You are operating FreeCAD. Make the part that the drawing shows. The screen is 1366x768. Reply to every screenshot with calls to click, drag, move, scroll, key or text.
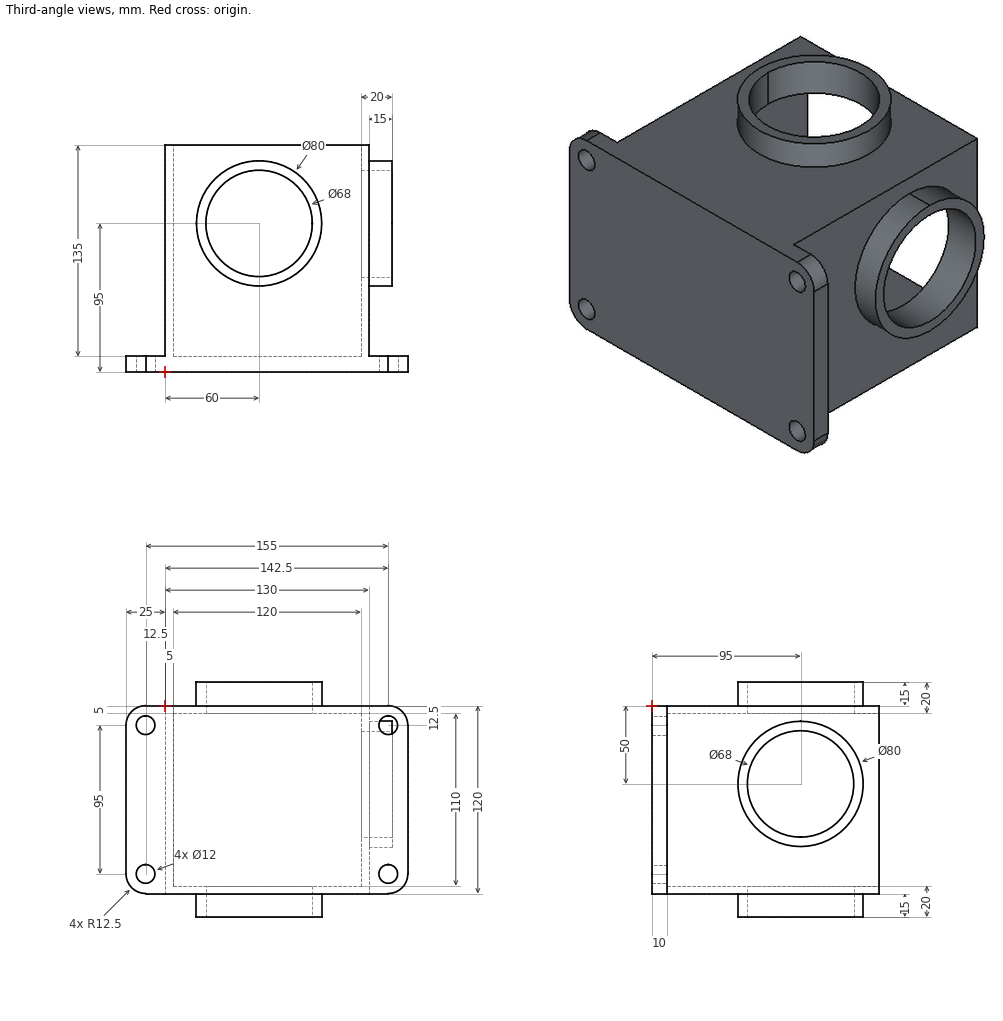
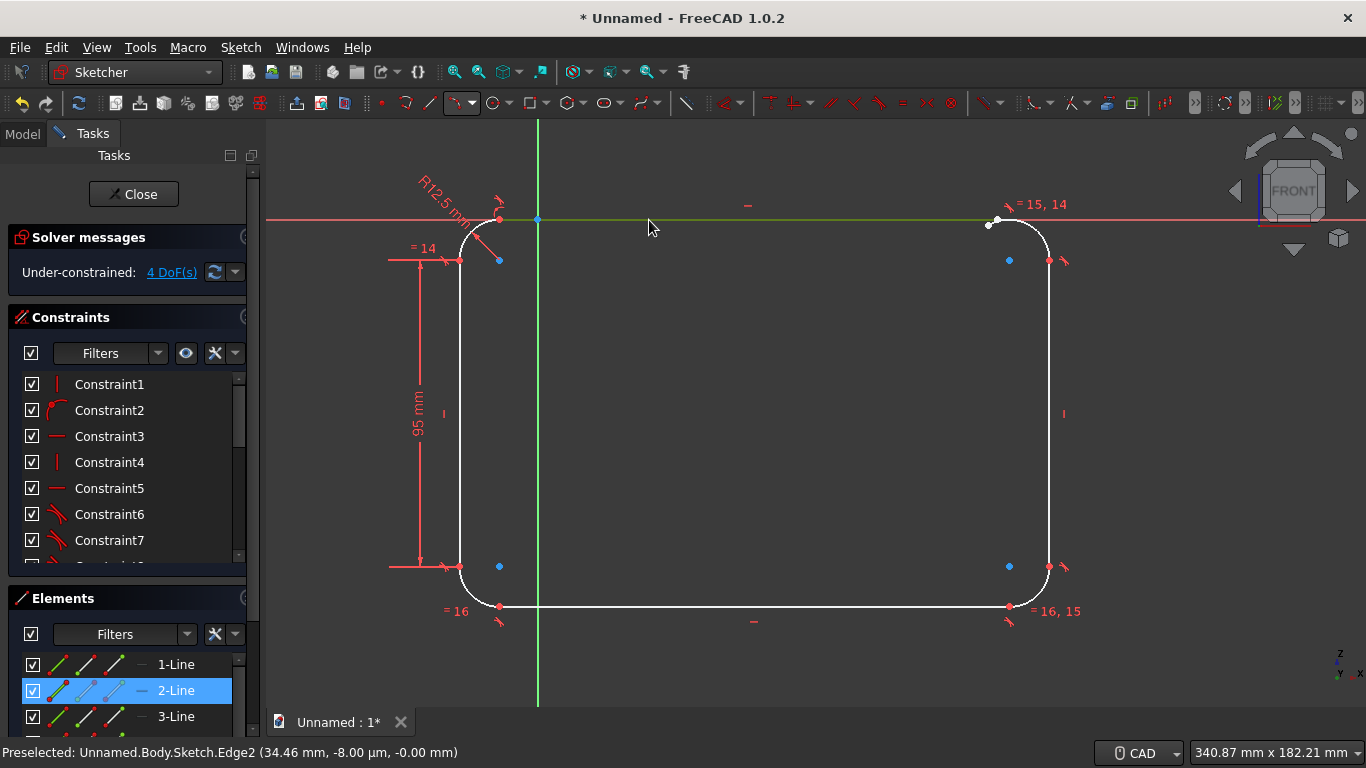
click(742, 104)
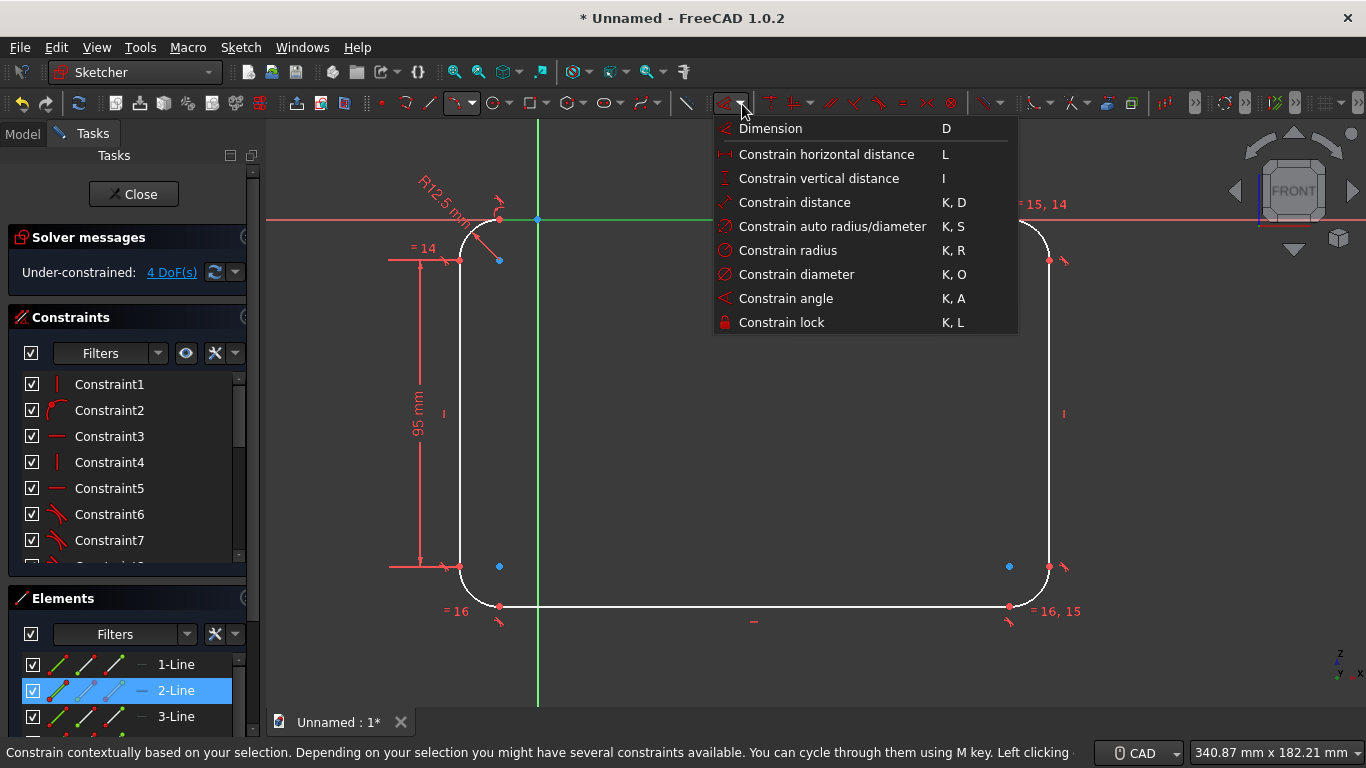
click(866, 154)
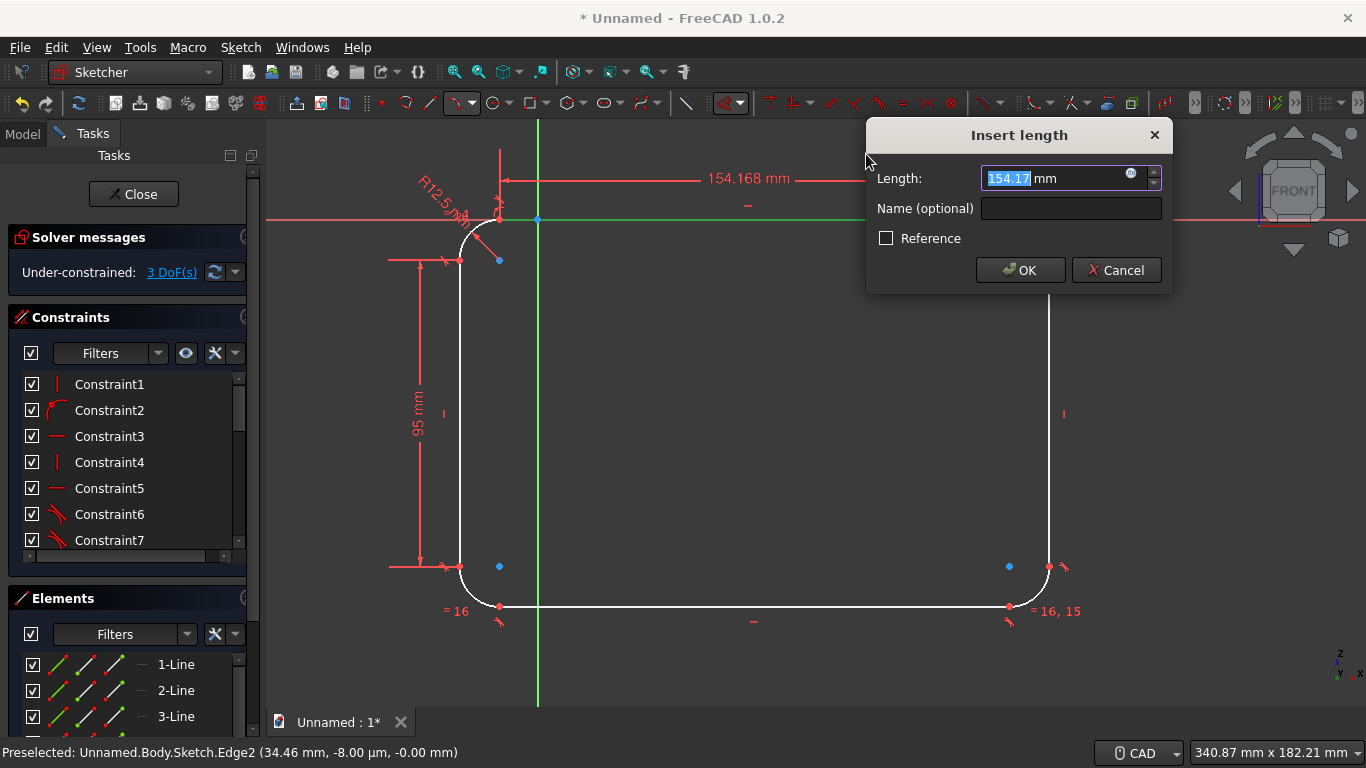
text(155)
key(Return)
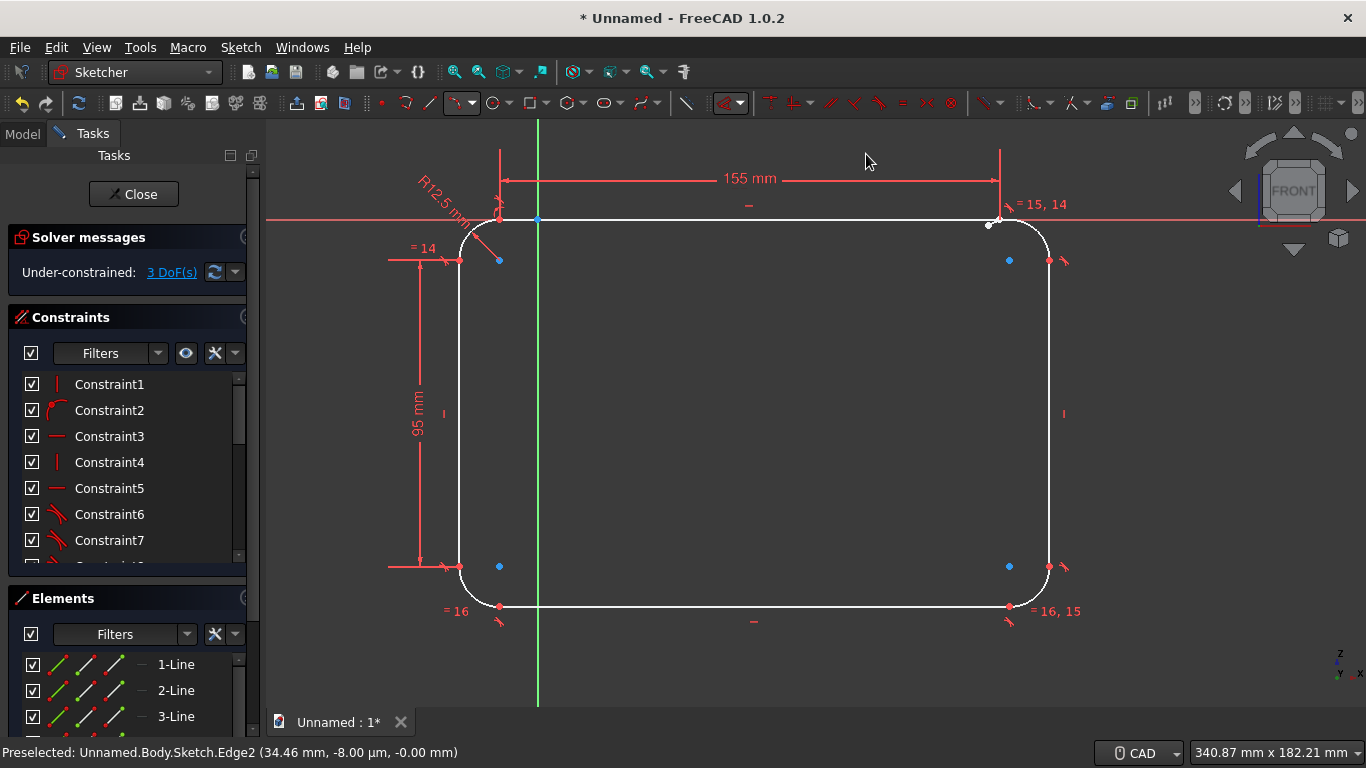
click(856, 607)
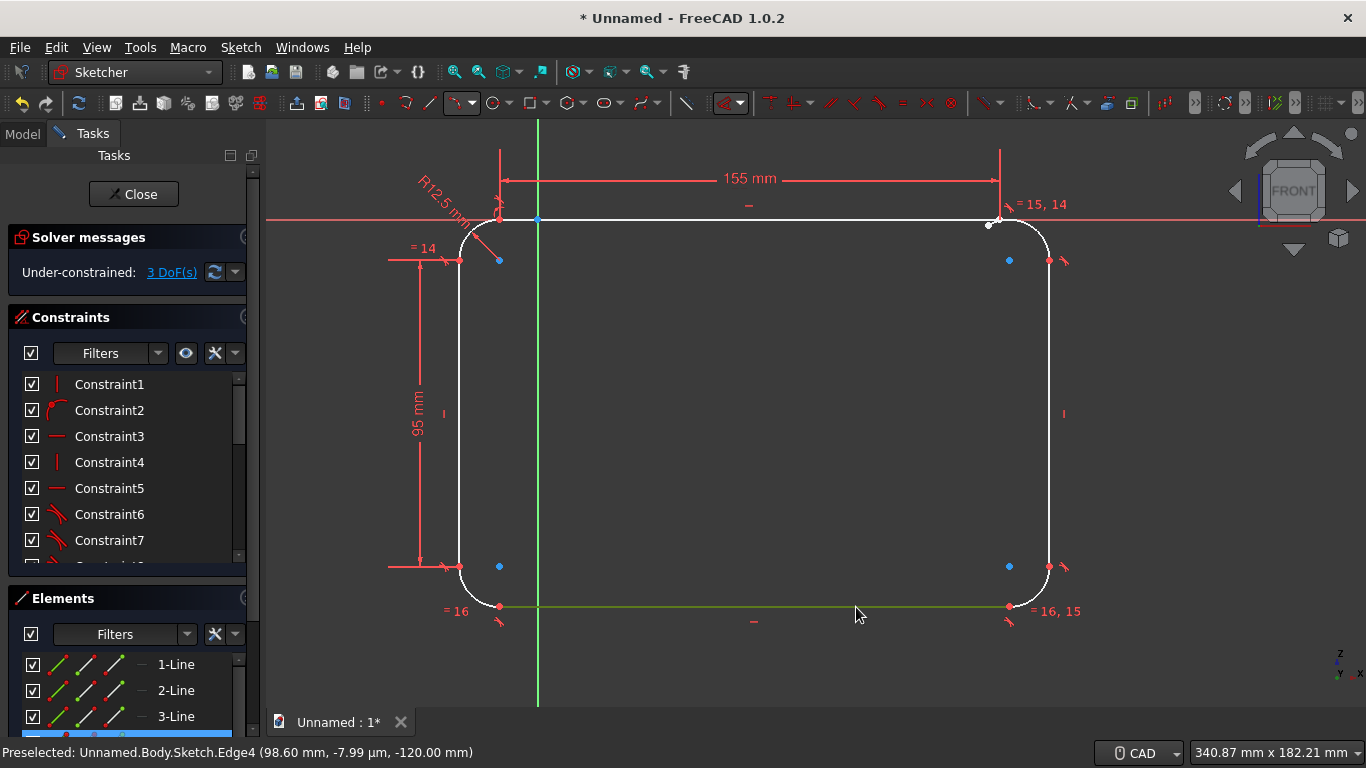
key(l)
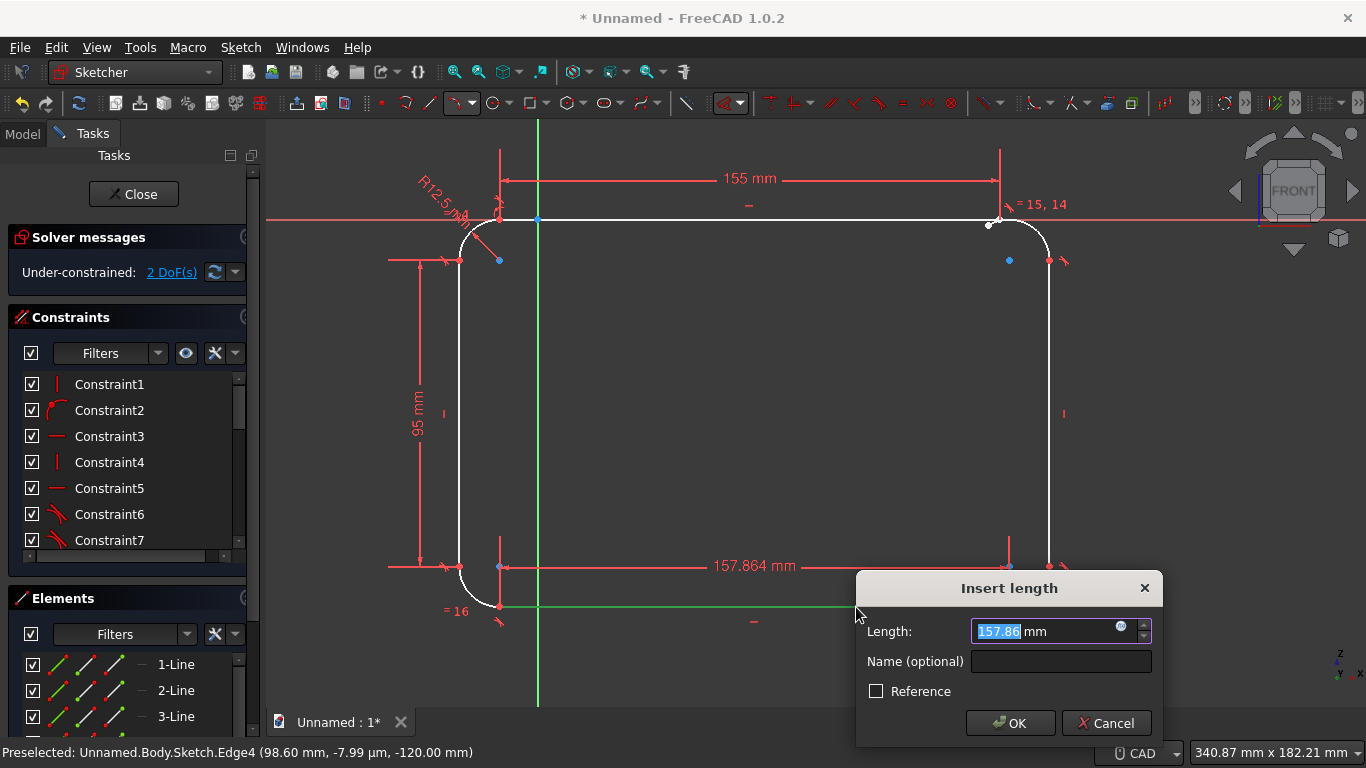
text(155)
key(Return)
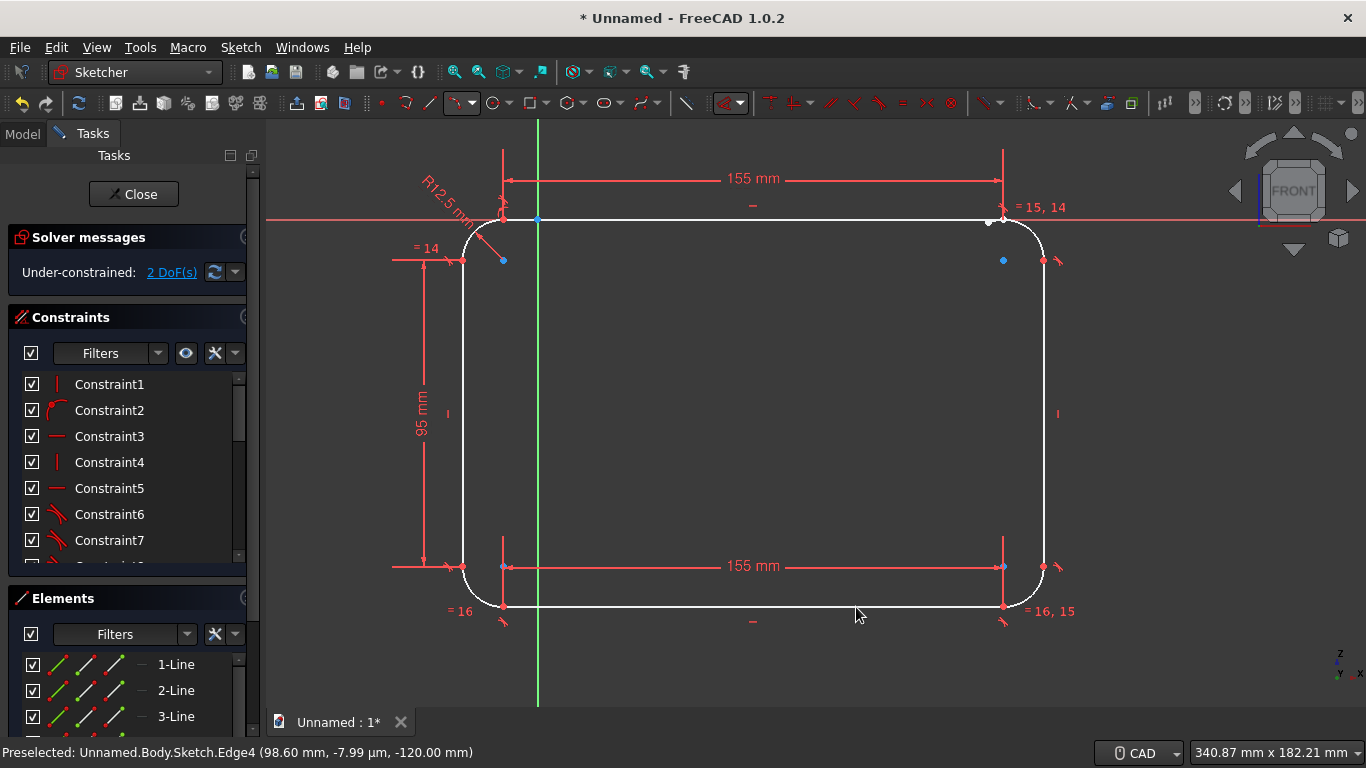
click(463, 567)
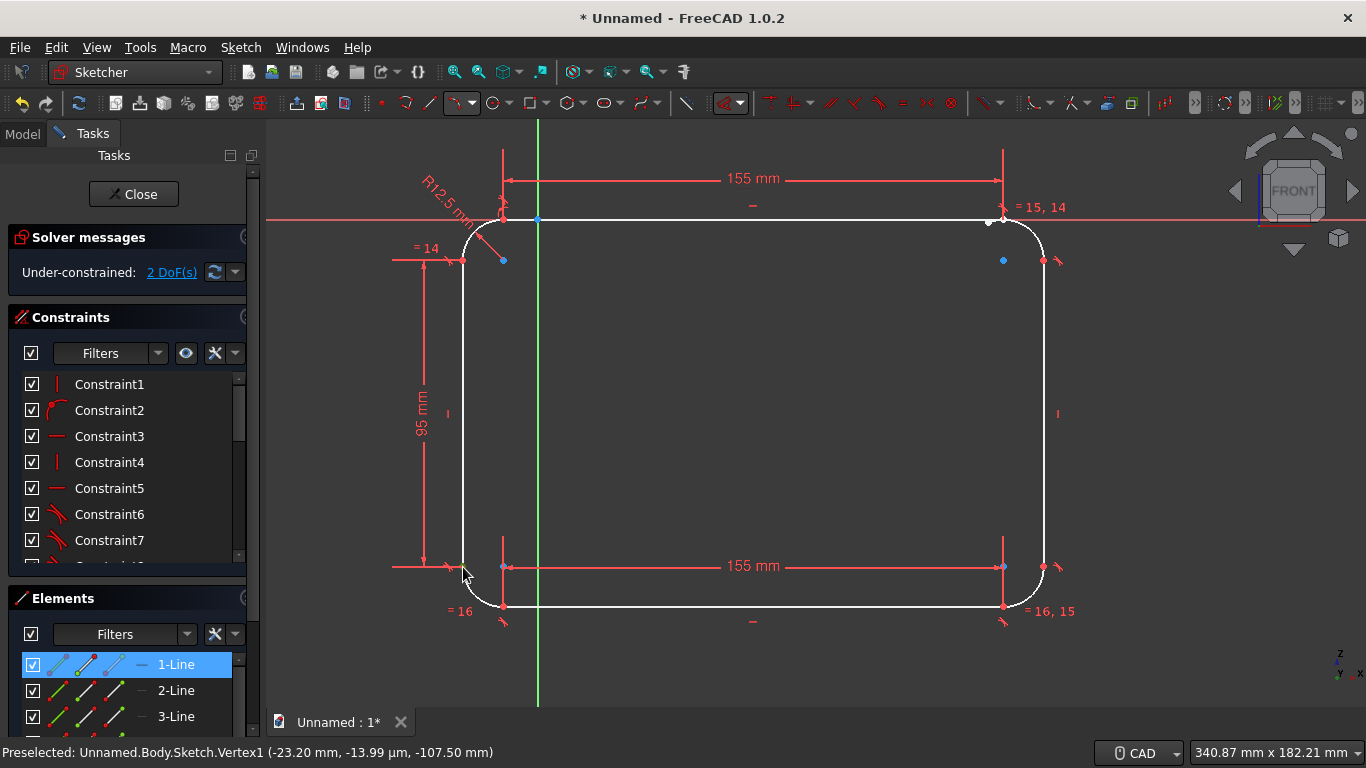
key(l)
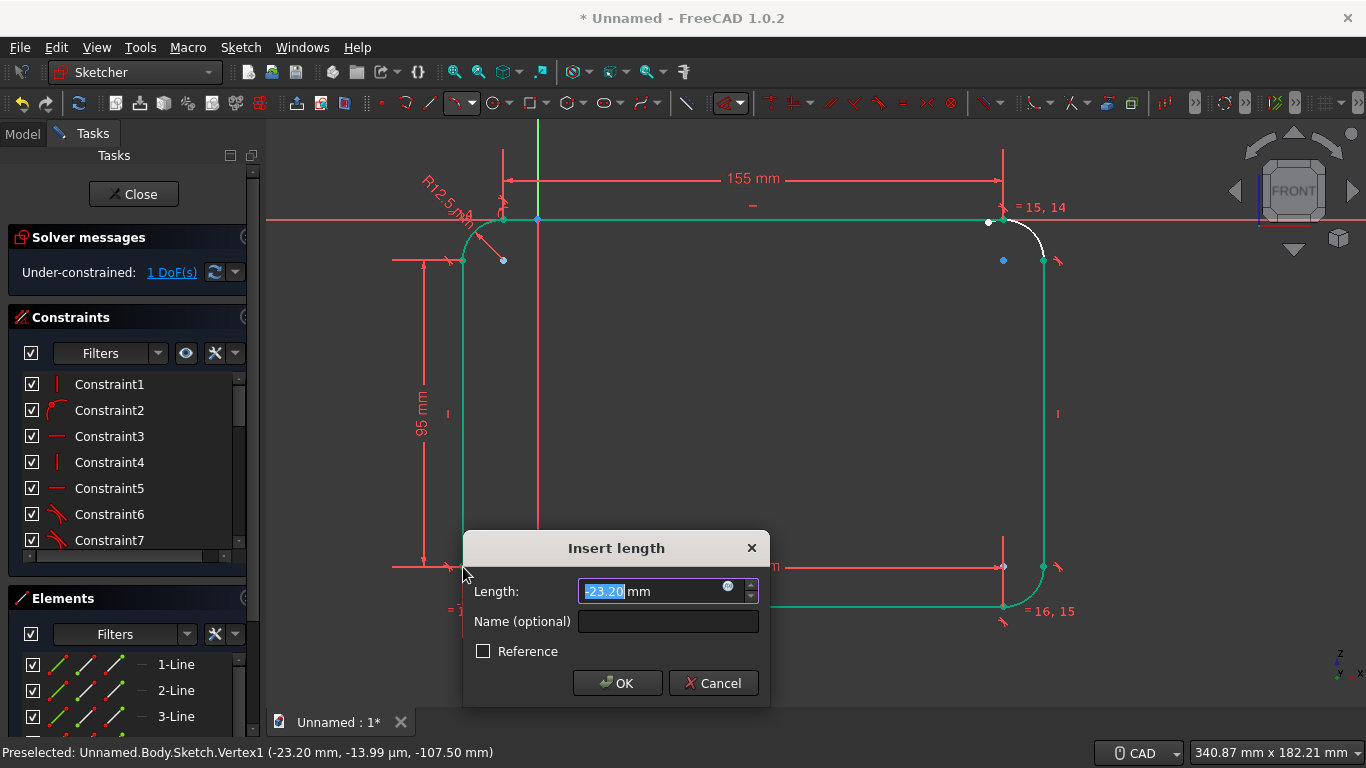
text(-25)
key(Return)